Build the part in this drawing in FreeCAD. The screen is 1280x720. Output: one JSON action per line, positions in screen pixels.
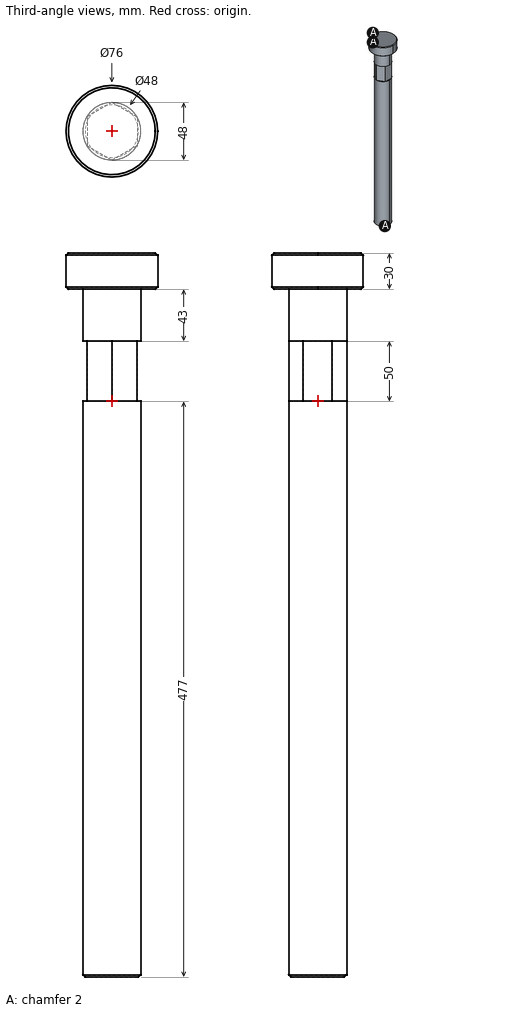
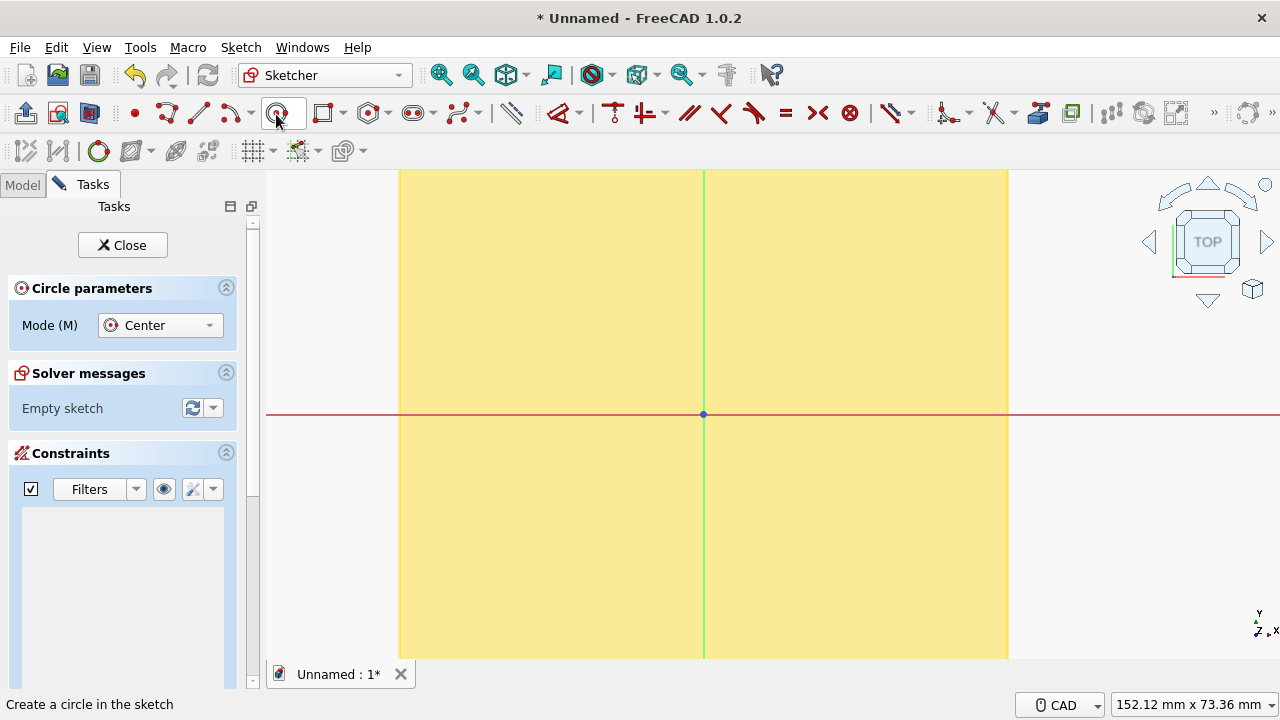
{"action": "left_click", "coordinate": [704, 414]}
{"action": "left_click", "coordinate": [817, 301]}
{"action": "key", "text": "Escape"}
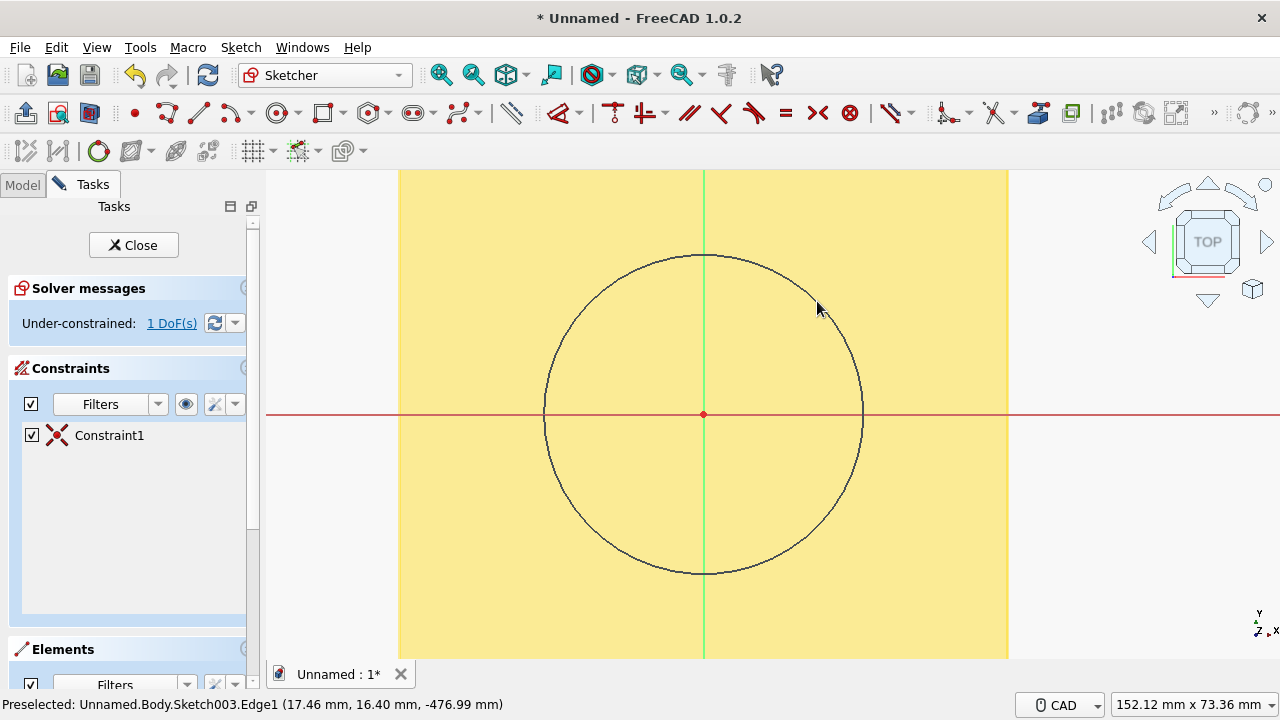
{"action": "left_click", "coordinate": [558, 114]}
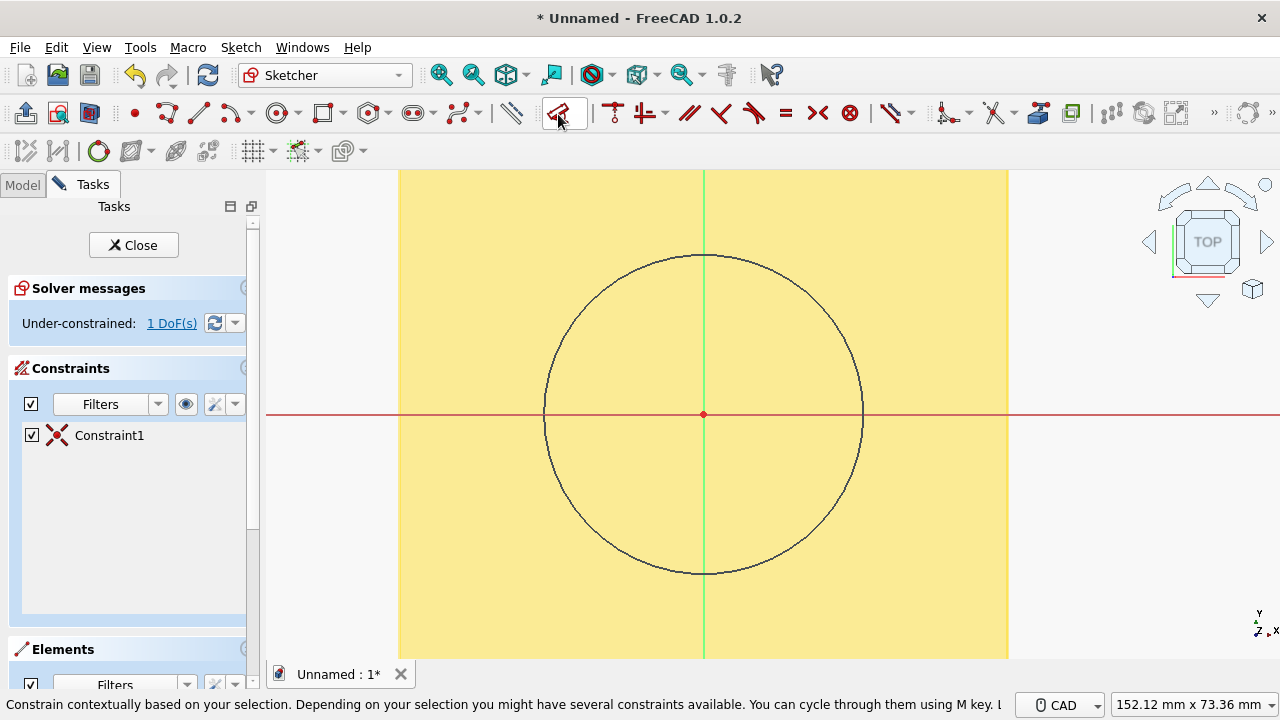
{"action": "left_click", "coordinate": [816, 301]}
{"action": "left_click", "coordinate": [839, 278]}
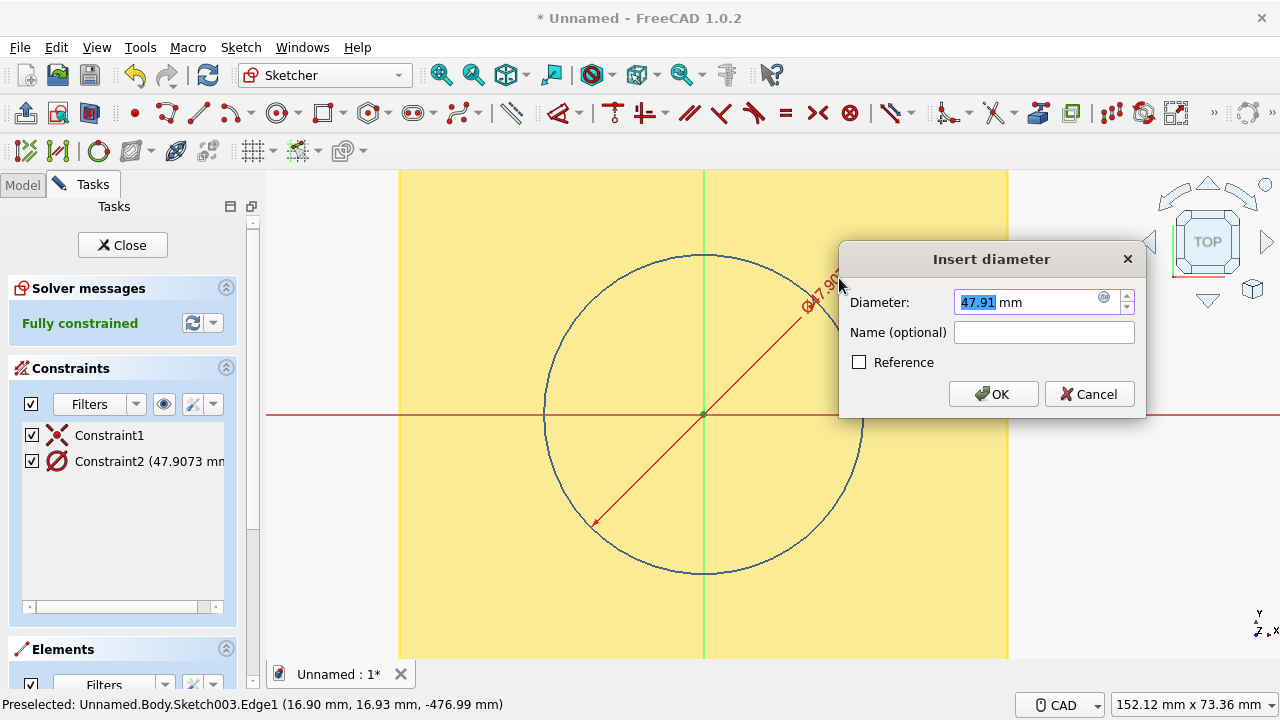
{"action": "type", "text": "48"}
{"action": "key", "text": "Return"}
{"action": "key", "text": "Escape"}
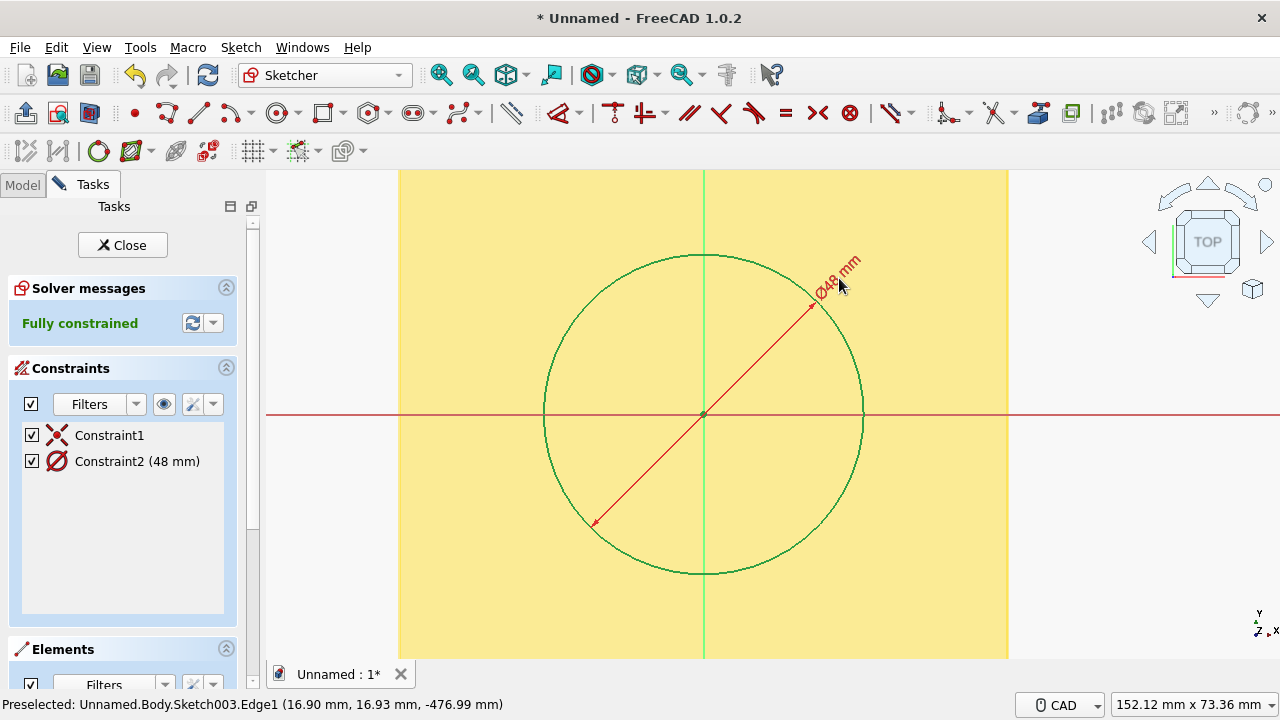
{"action": "left_click", "coordinate": [123, 245]}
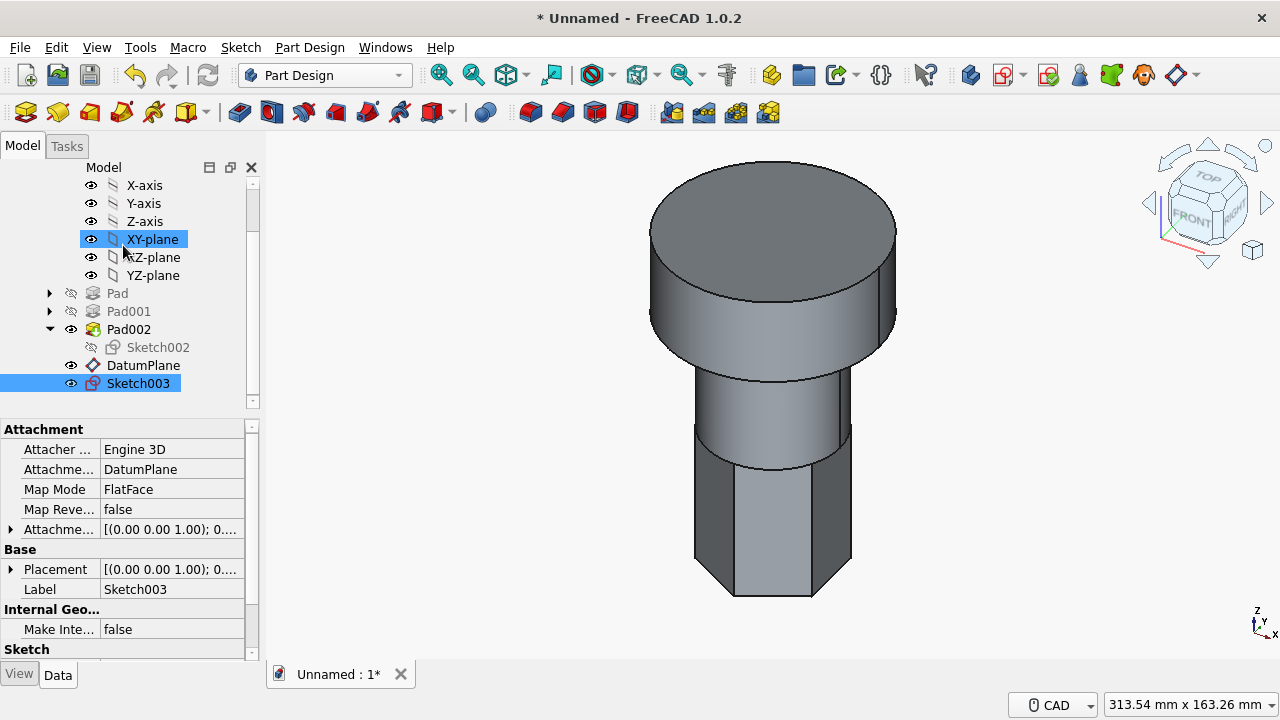
{"action": "left_click", "coordinate": [26, 112]}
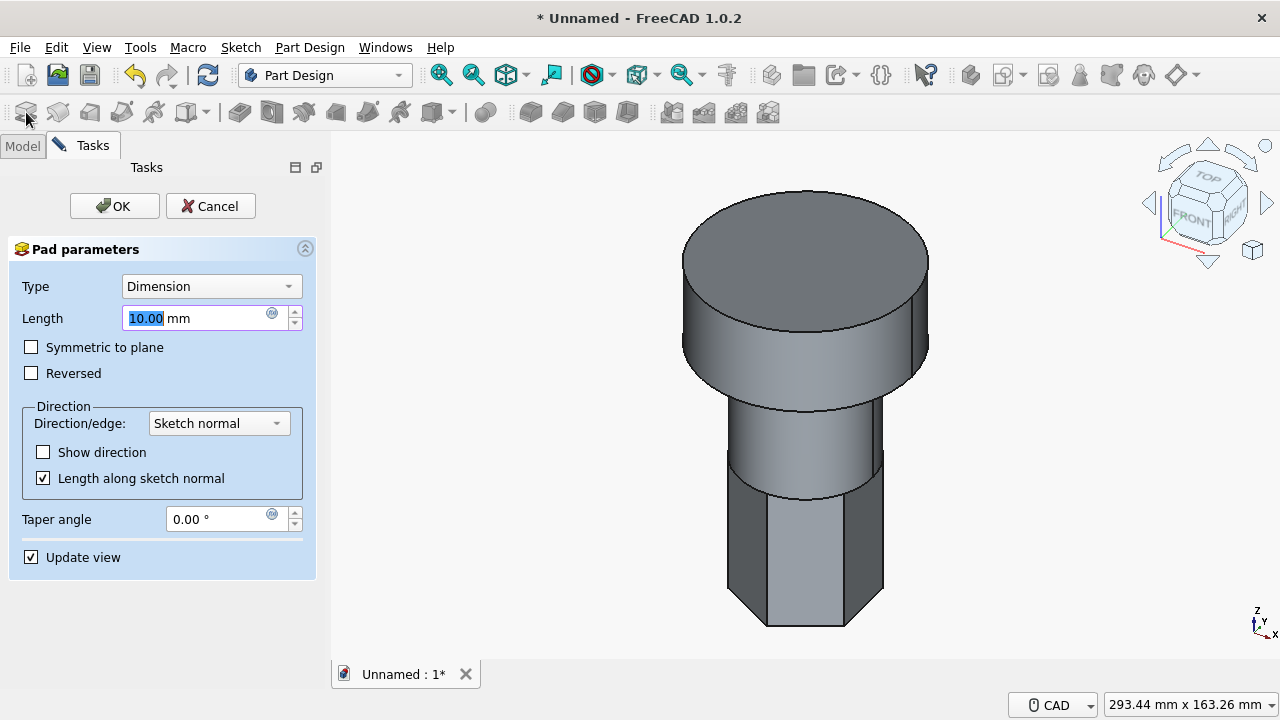
{"action": "type", "text": "477"}
{"action": "key", "text": "Tab"}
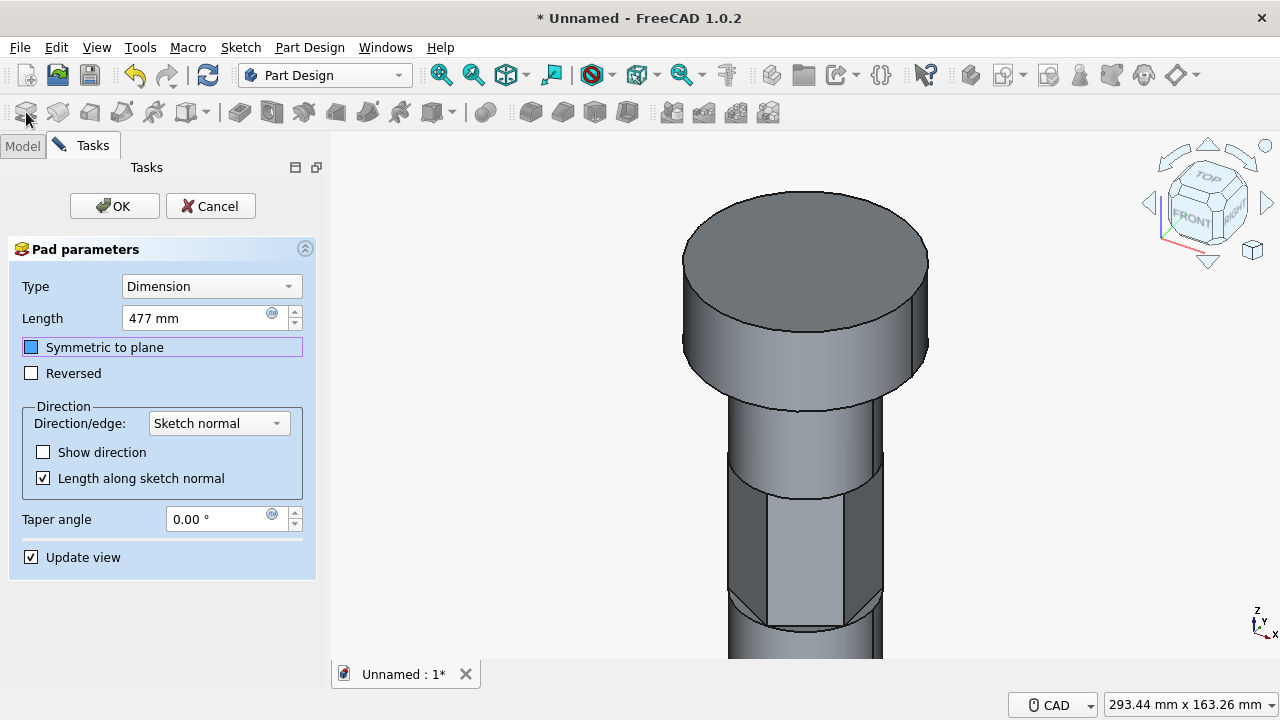
{"action": "left_click", "coordinate": [115, 206]}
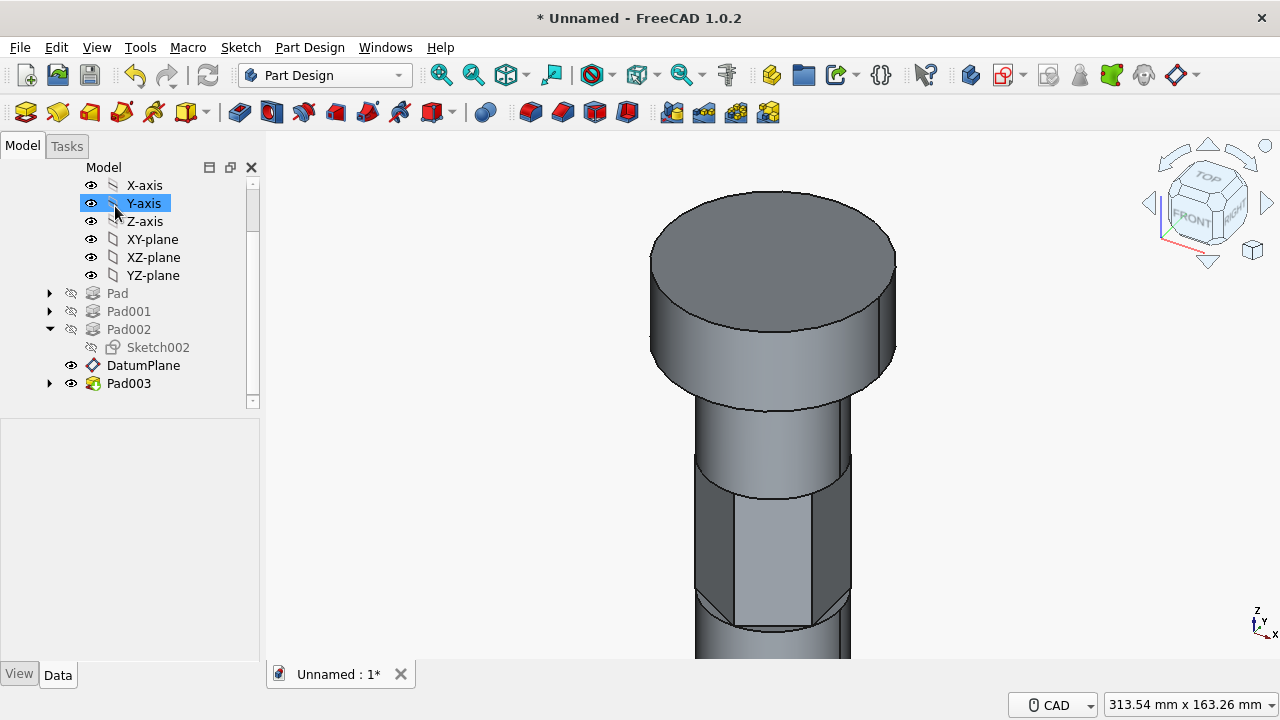
{"action": "left_click", "coordinate": [116, 365]}
{"action": "key", "text": "space"}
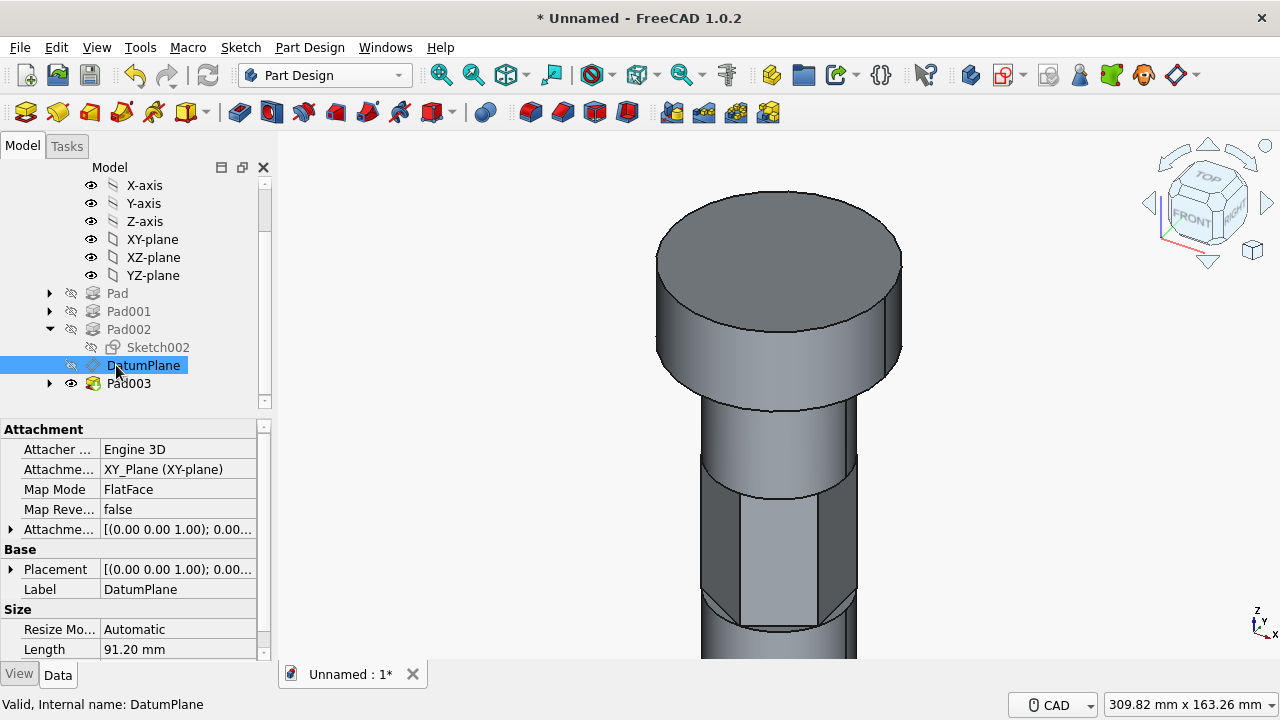
{"action": "left_click", "coordinate": [442, 76]}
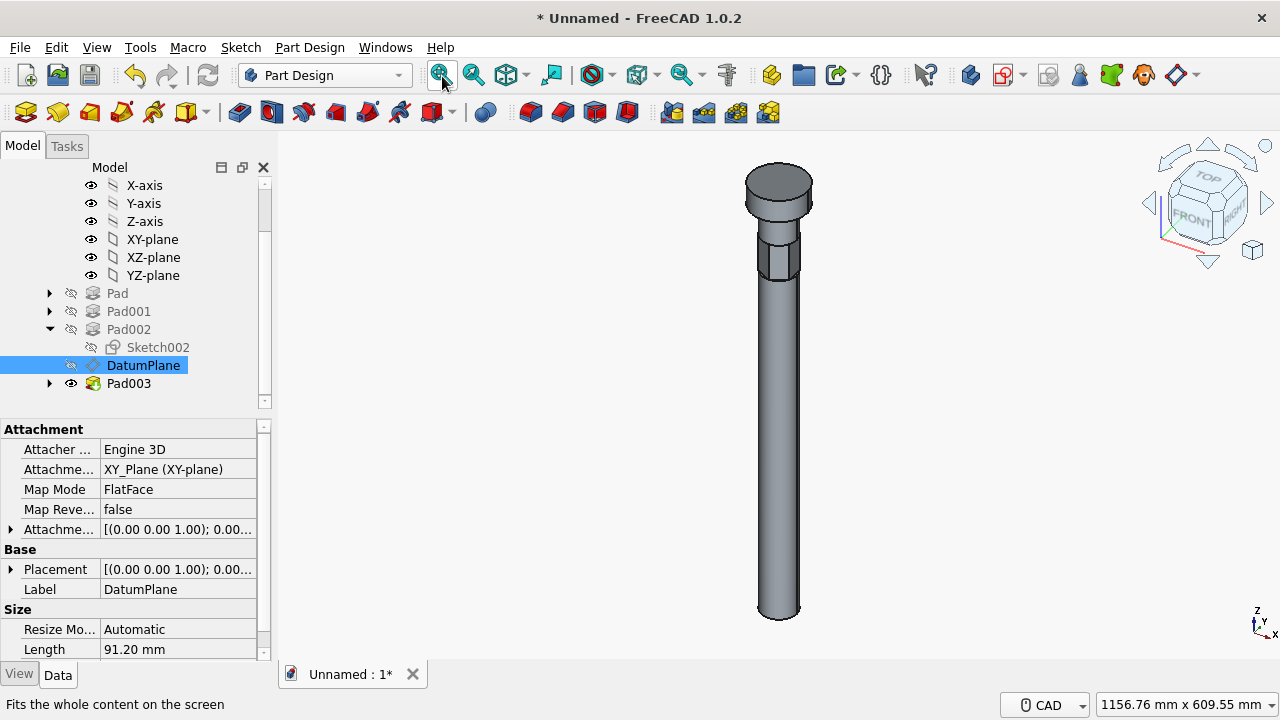
{"action": "left_click", "coordinate": [746, 183]}